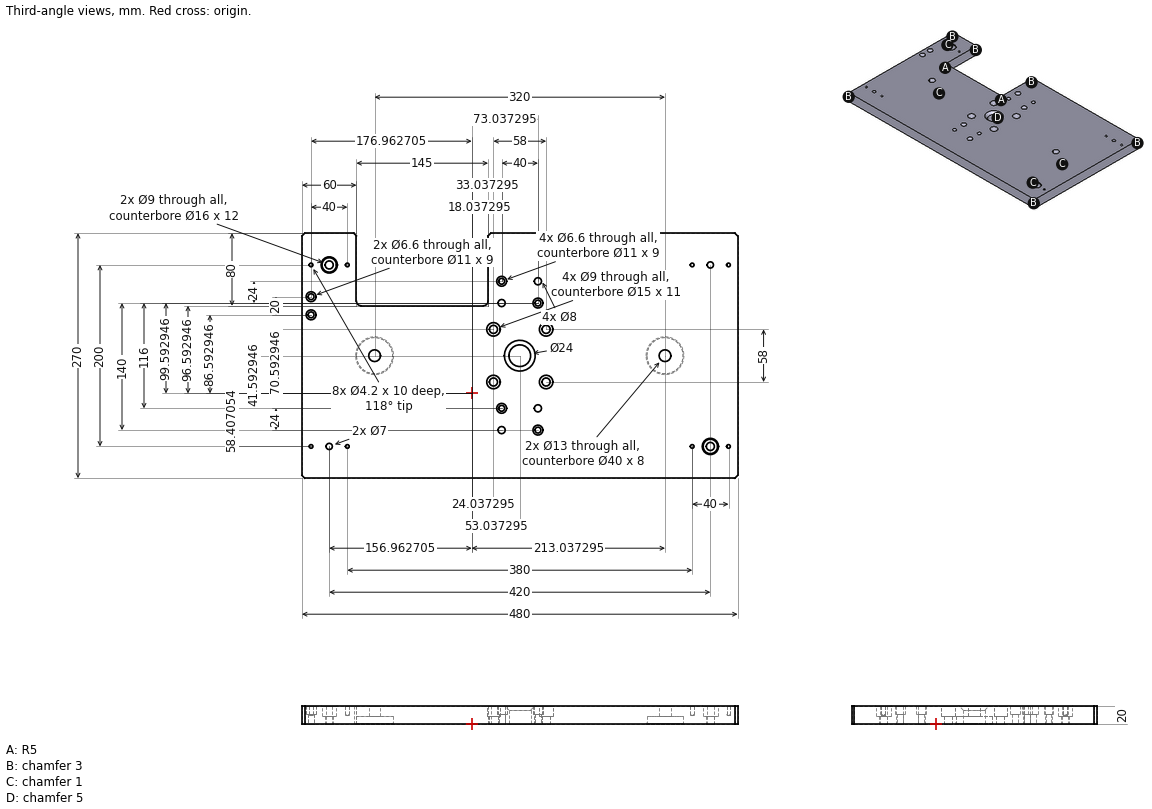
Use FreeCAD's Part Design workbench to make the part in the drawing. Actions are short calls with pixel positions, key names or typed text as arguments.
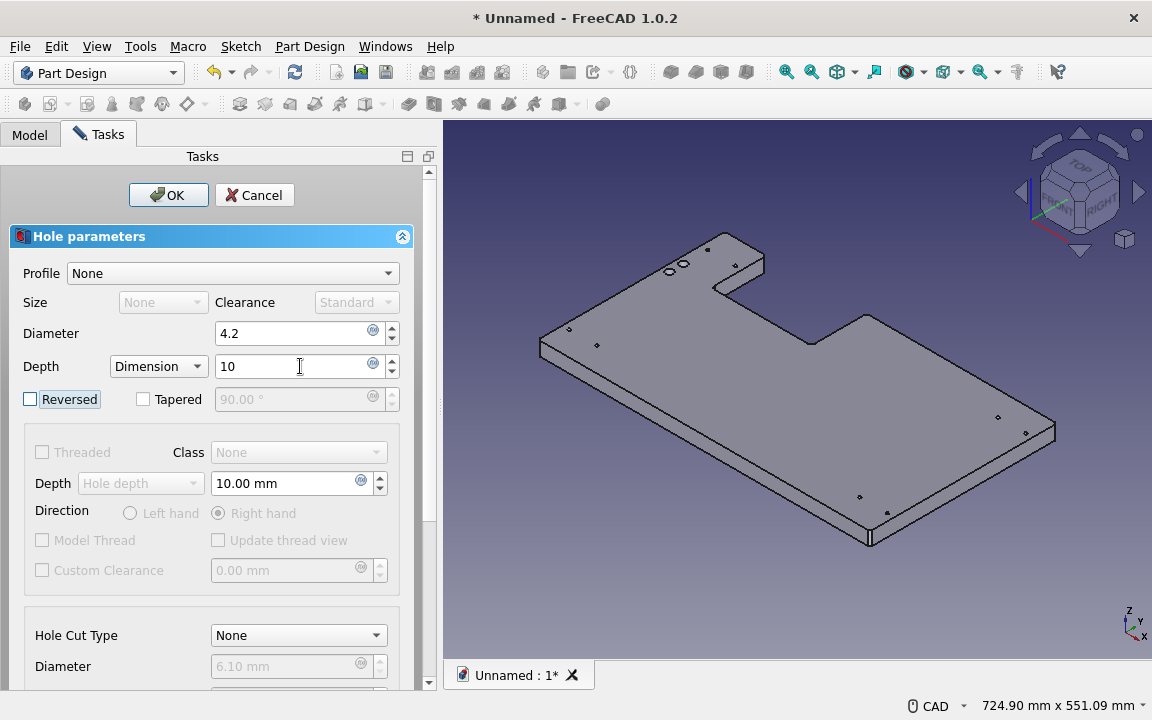
click(169, 195)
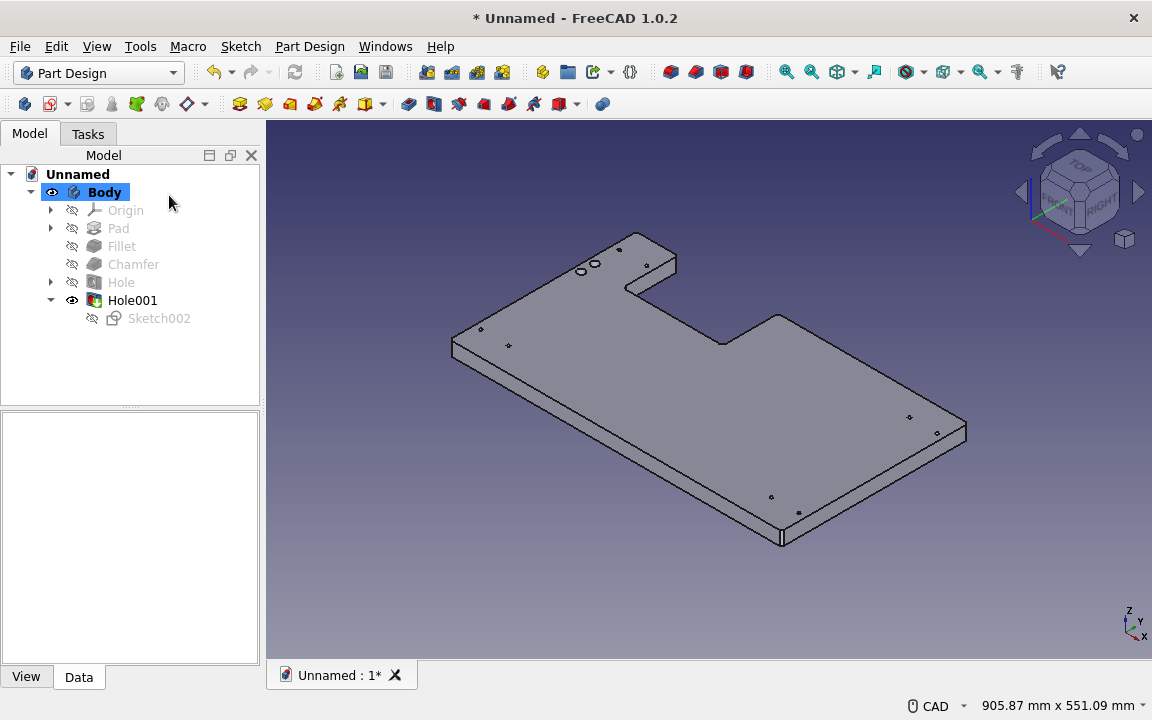
click(756, 408)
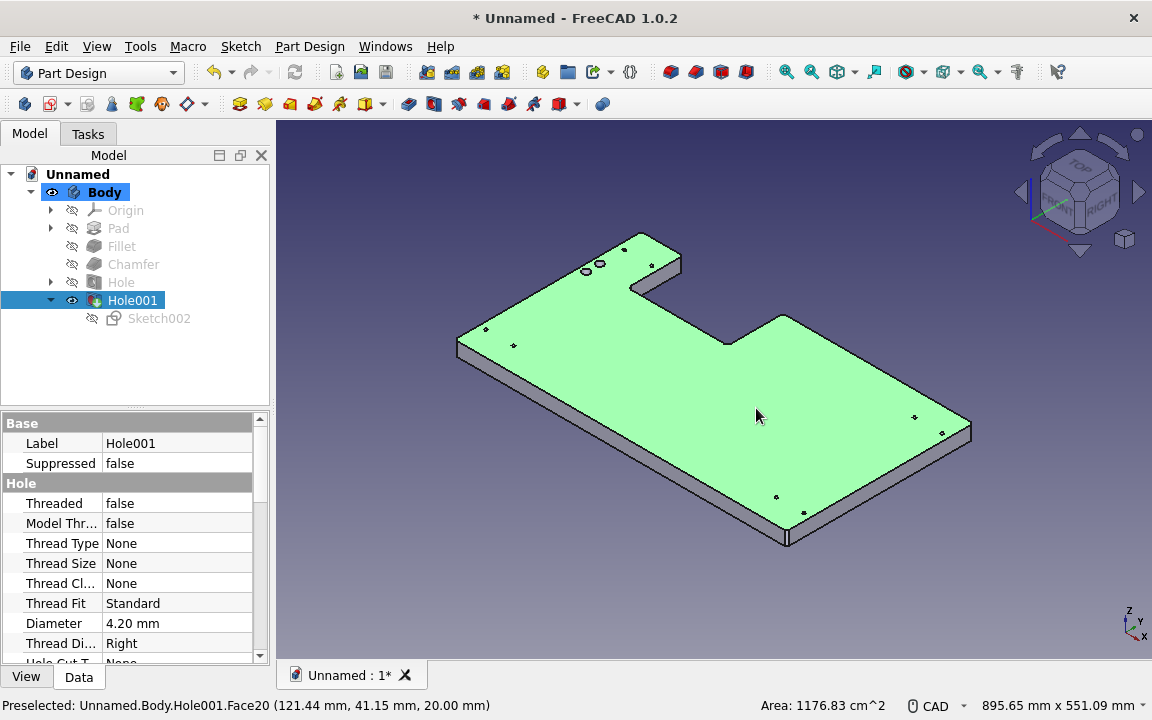
click(50, 104)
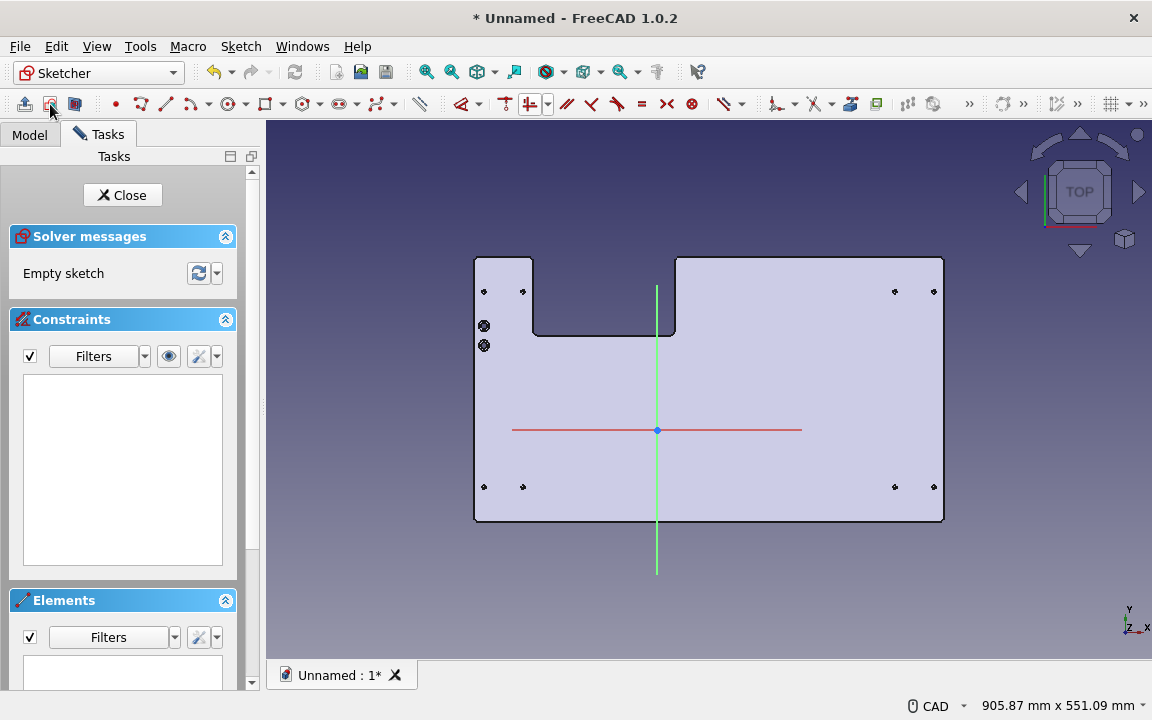
key(g)
key(c)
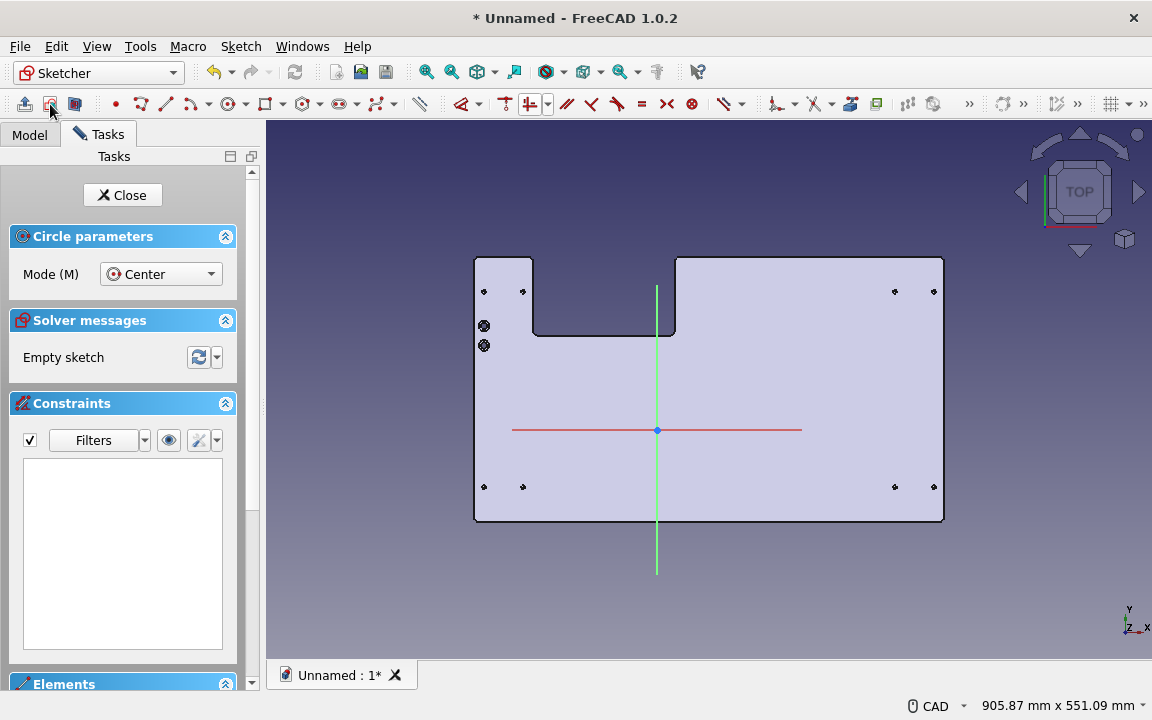
scroll(504, 487, up, 10)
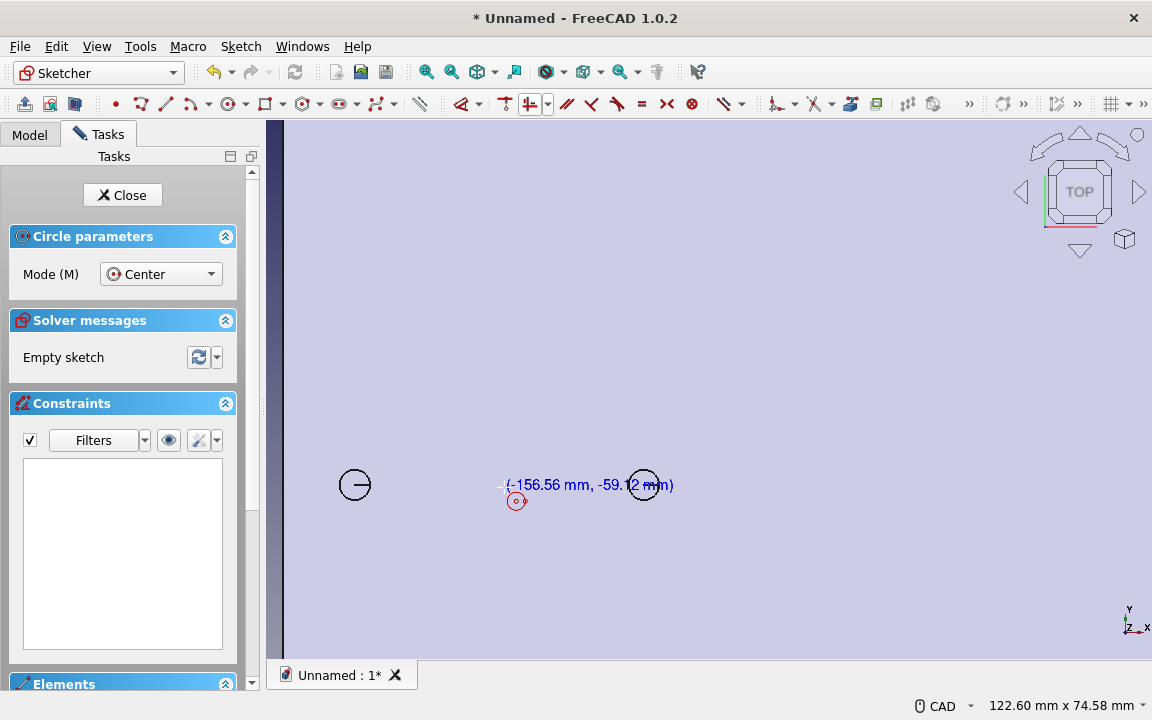
scroll(368, 514, down, 9)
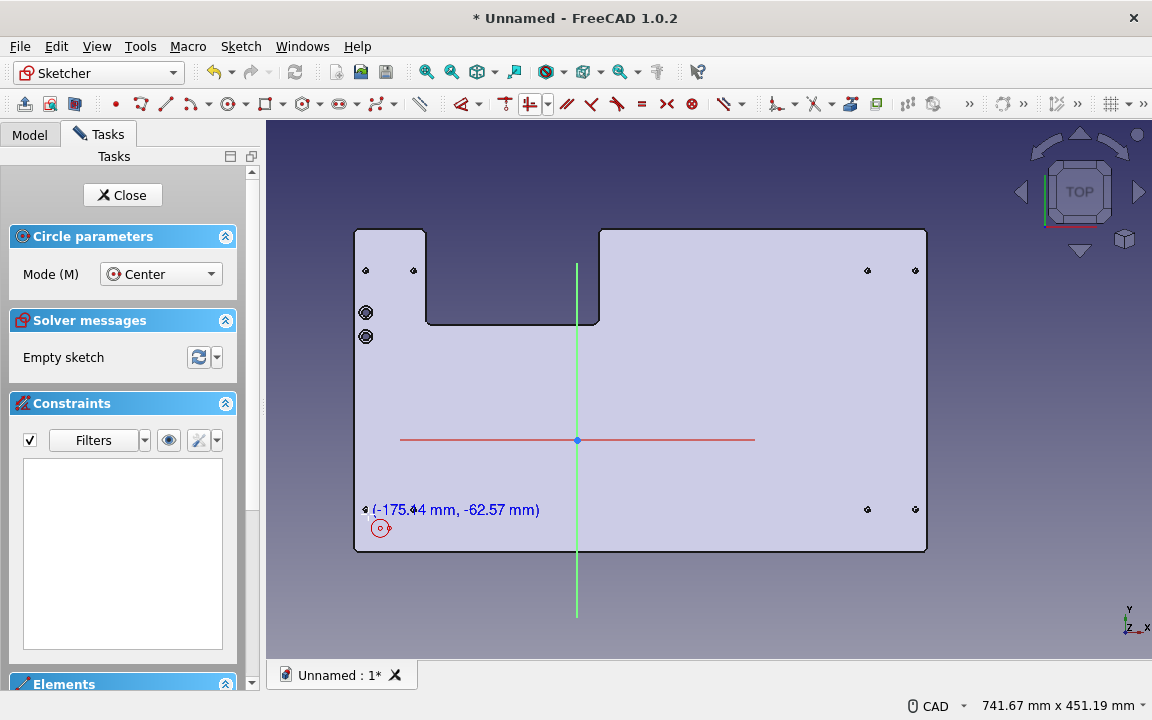
click(390, 510)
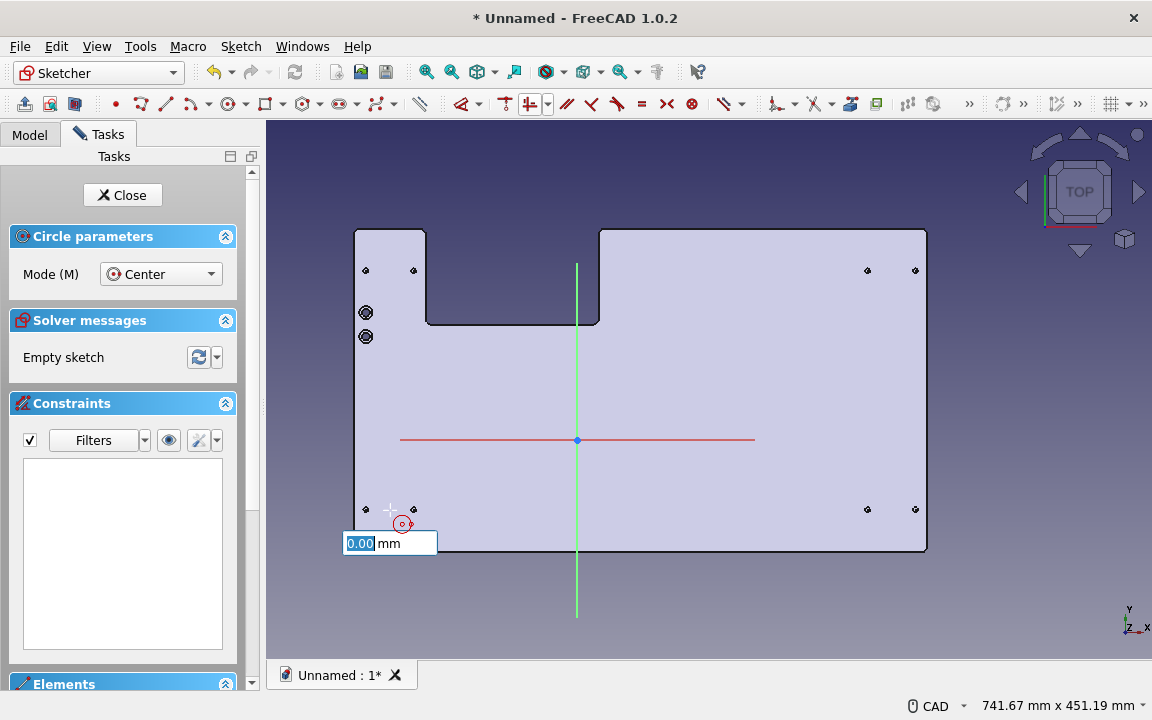
scroll(393, 507, up, 7)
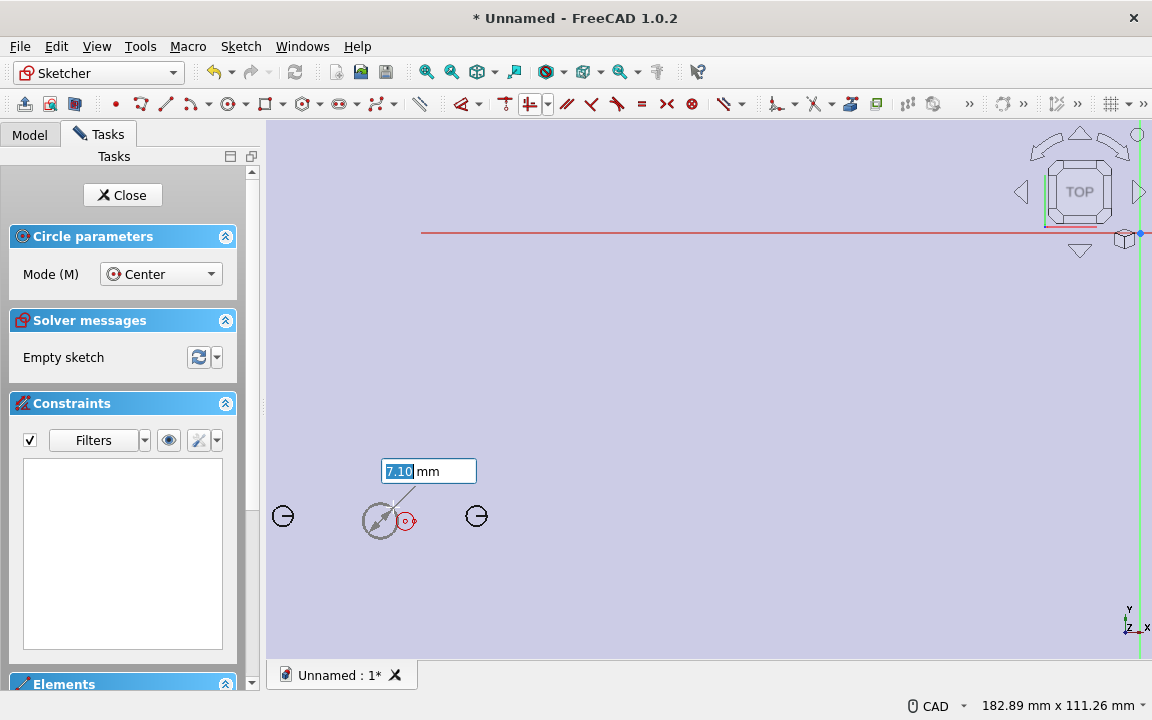
click(392, 504)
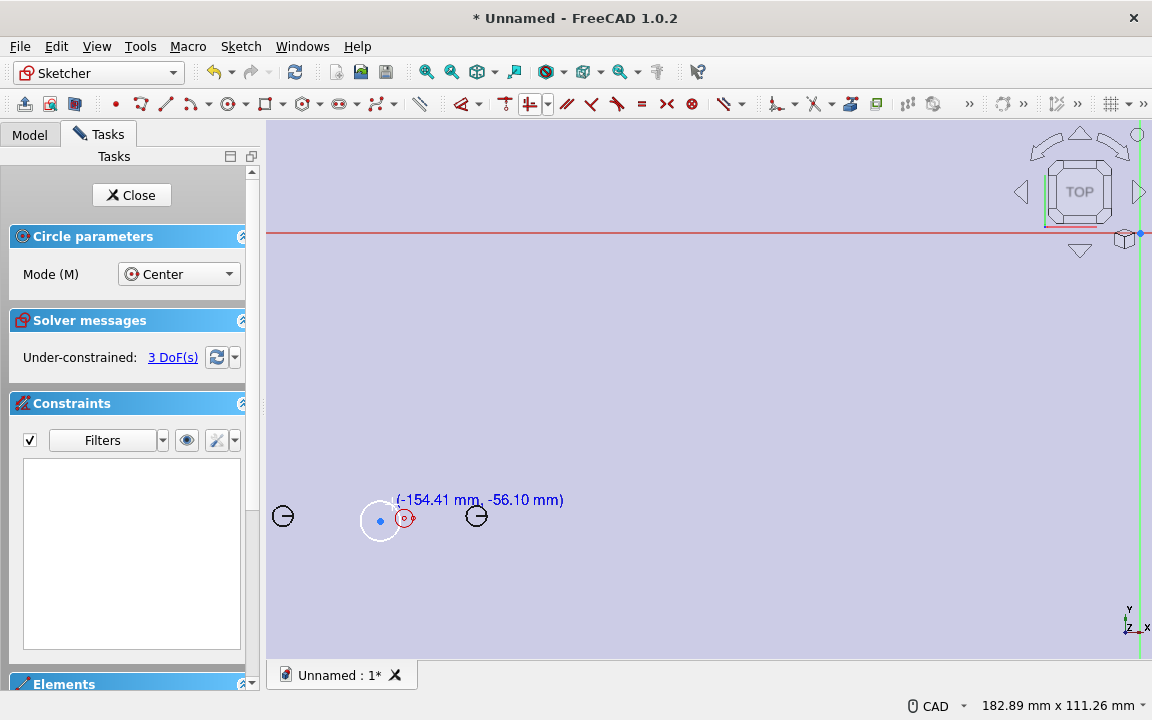
scroll(393, 507, down, 7)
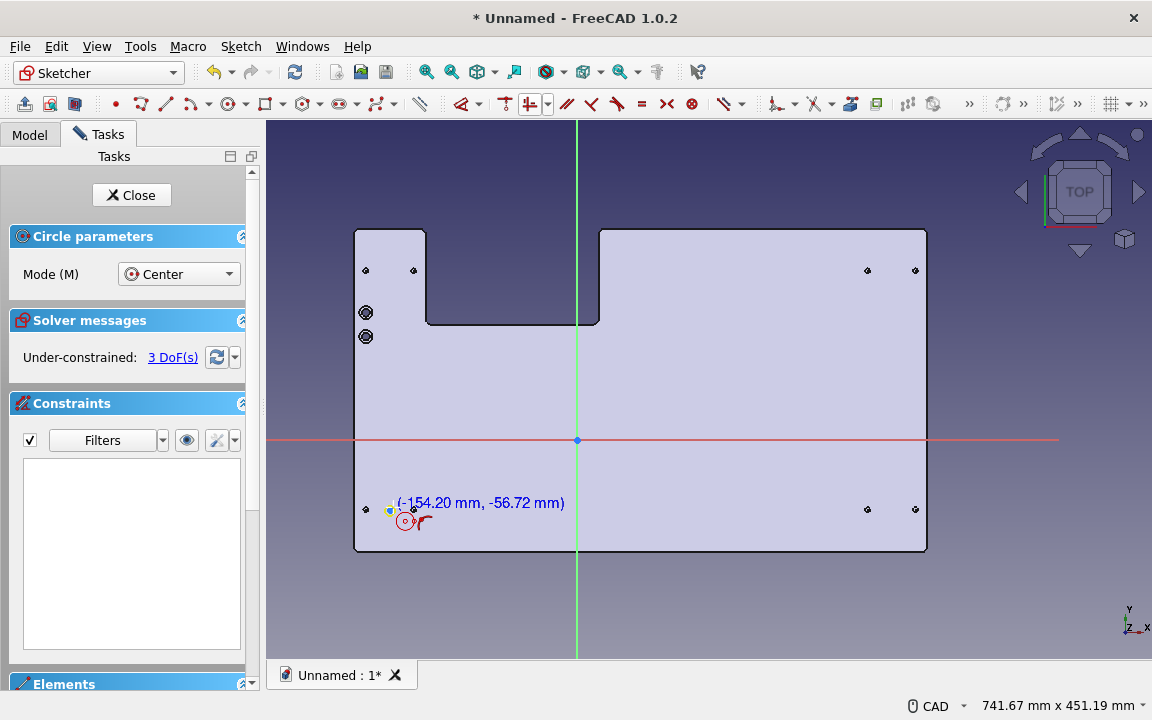
scroll(892, 271, up, 9)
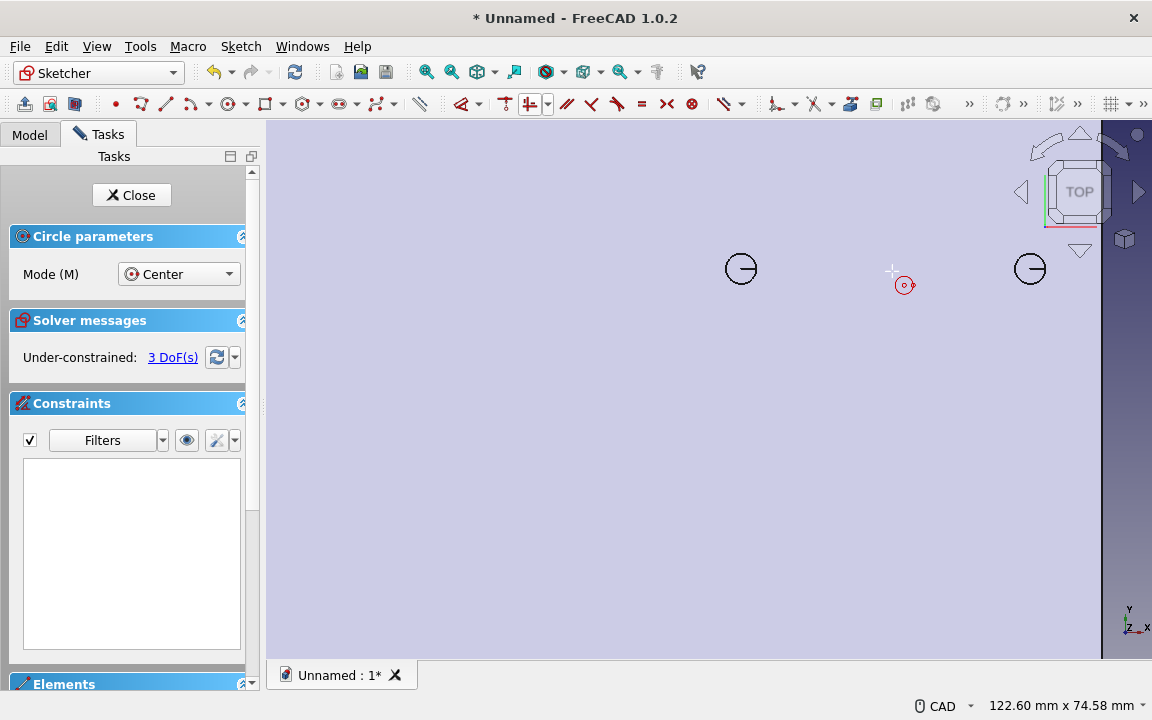
scroll(892, 270, down, 9)